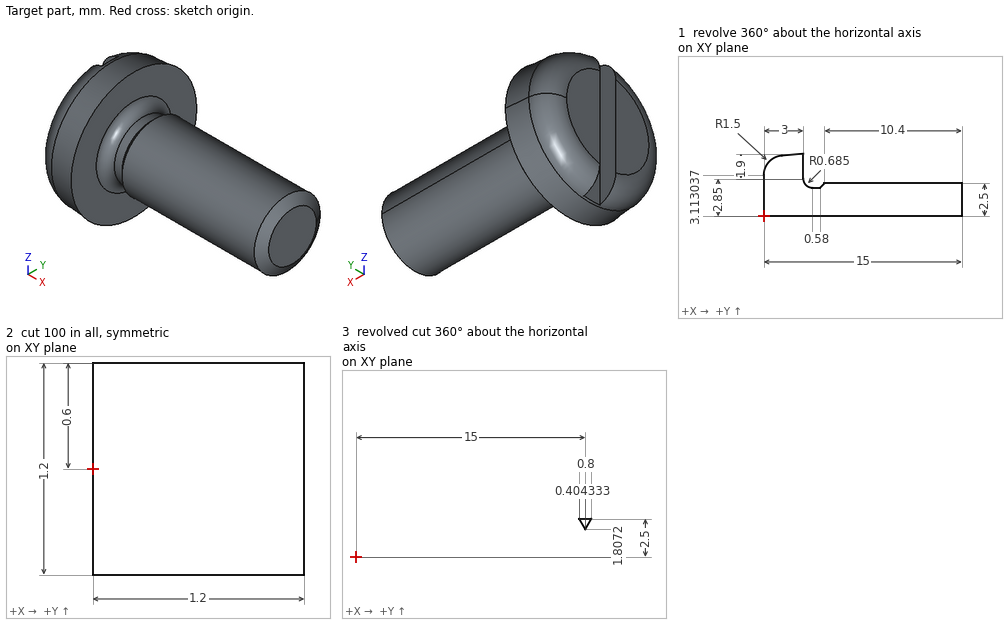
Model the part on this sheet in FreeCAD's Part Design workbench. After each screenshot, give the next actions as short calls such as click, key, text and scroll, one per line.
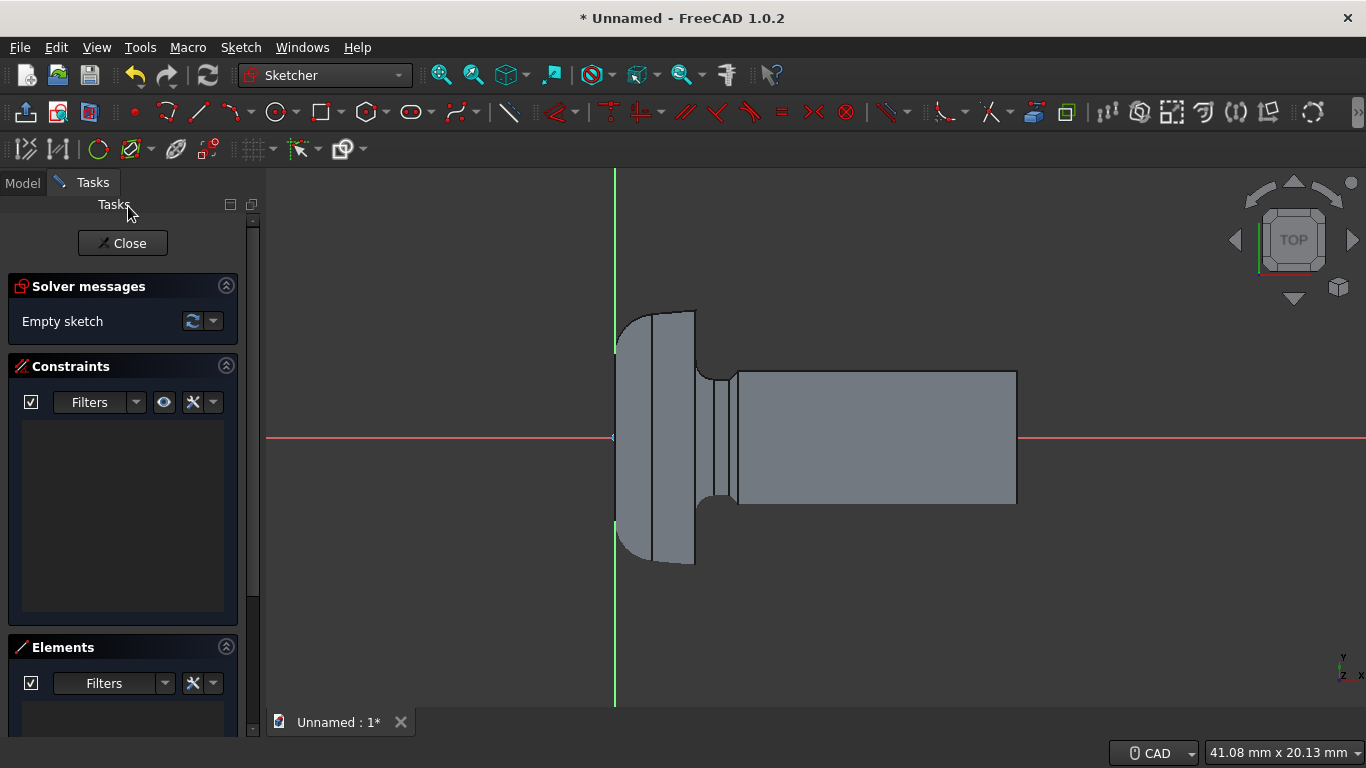
click(90, 112)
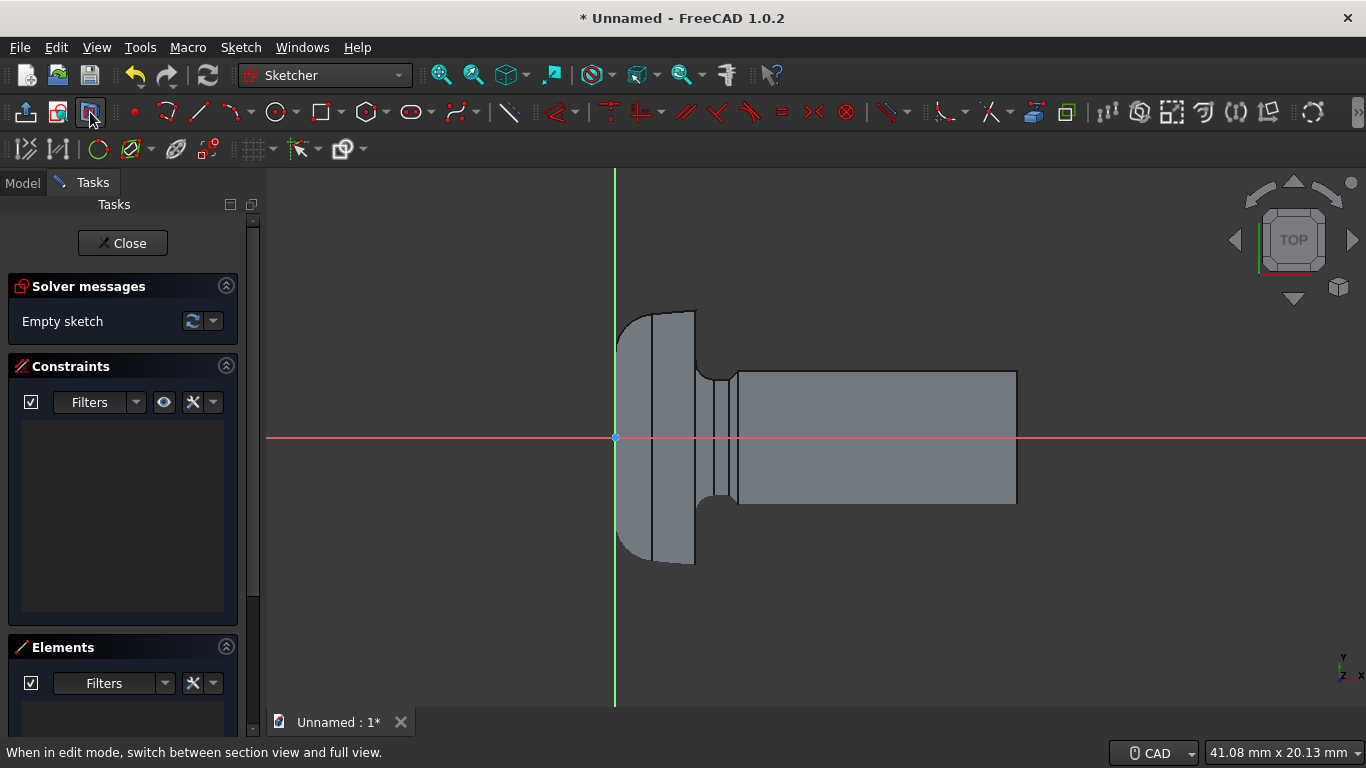
scroll(620, 438, up, 12)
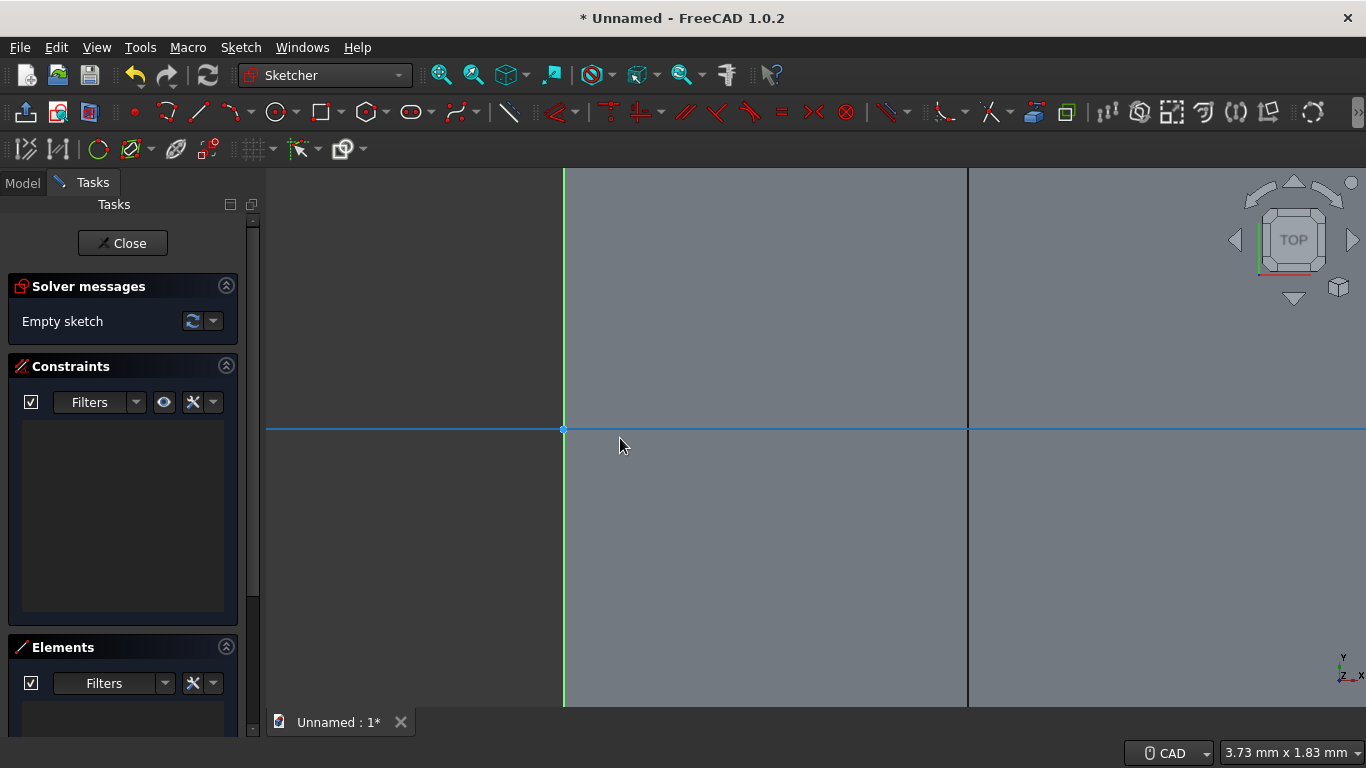
key(g)
key(r)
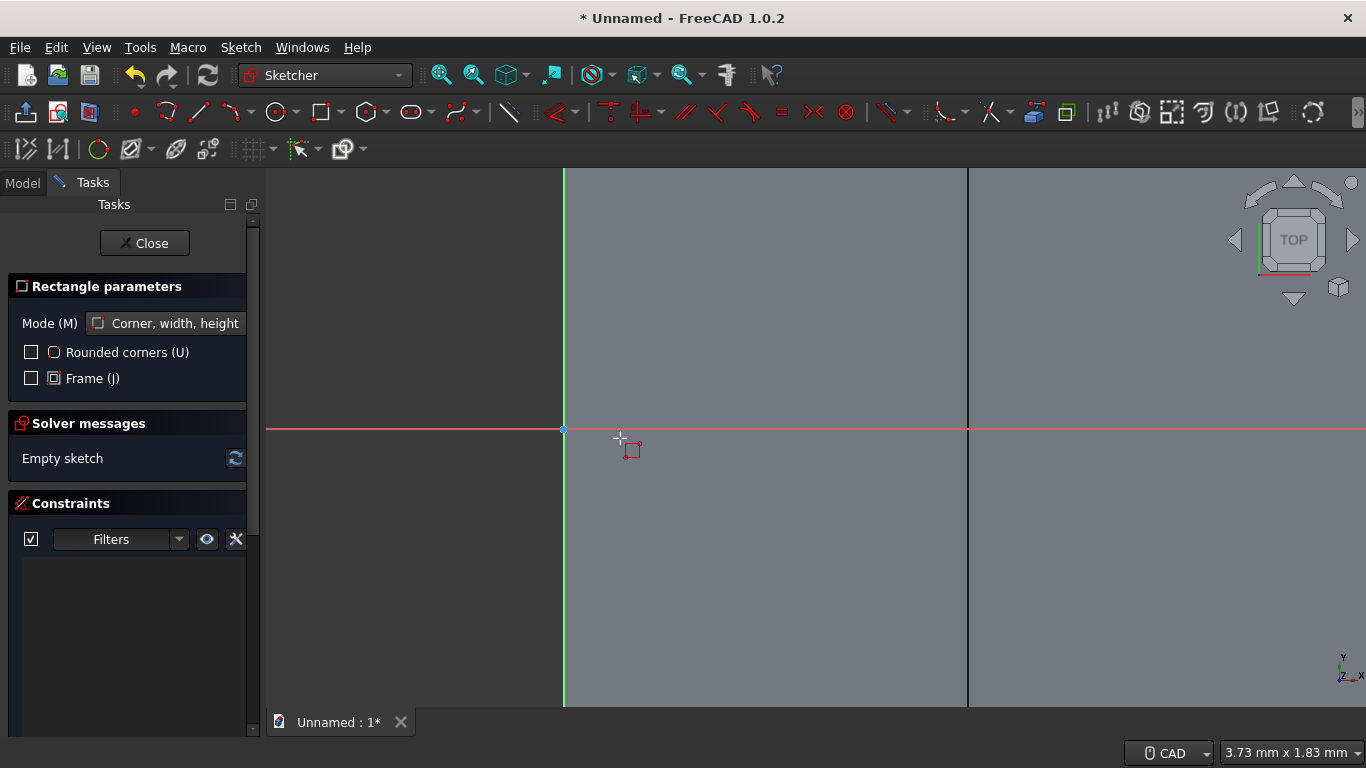
click(564, 252)
click(918, 606)
key(Escape)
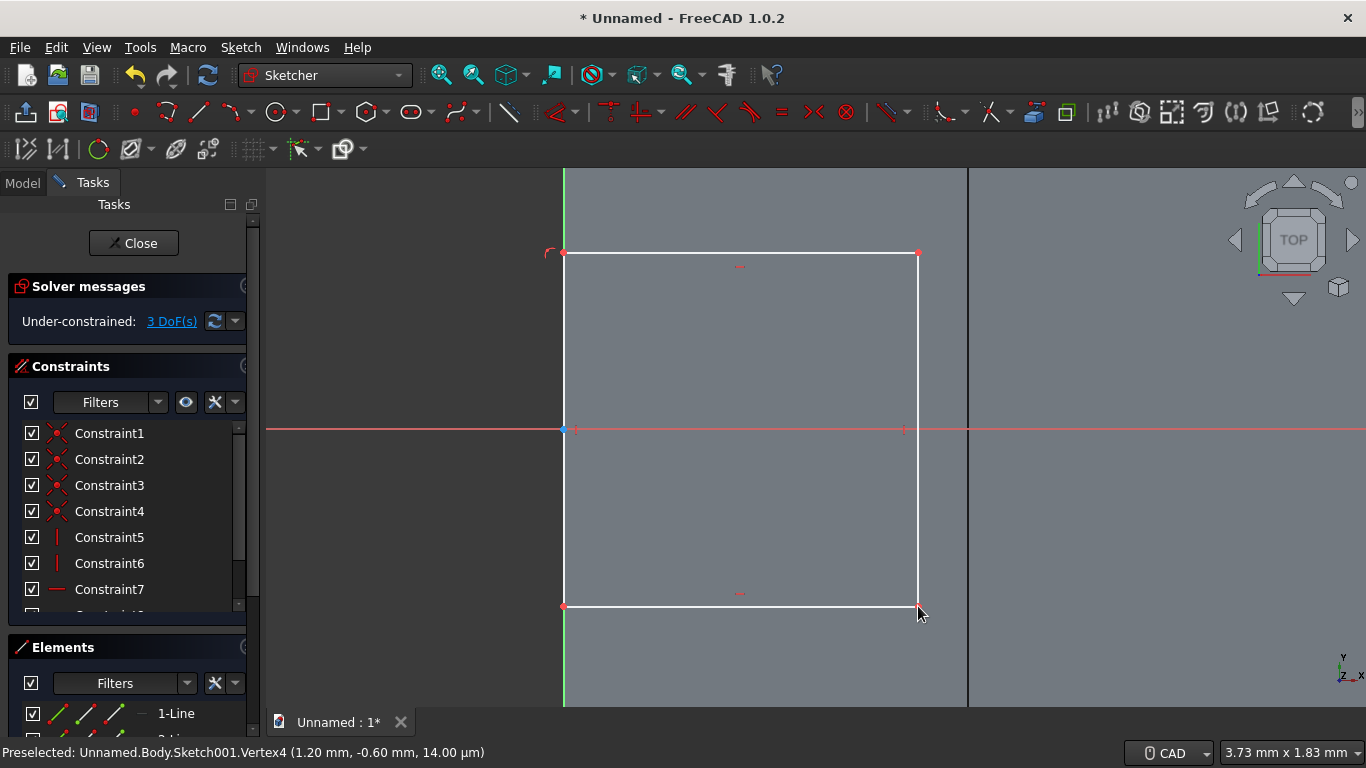
key(d)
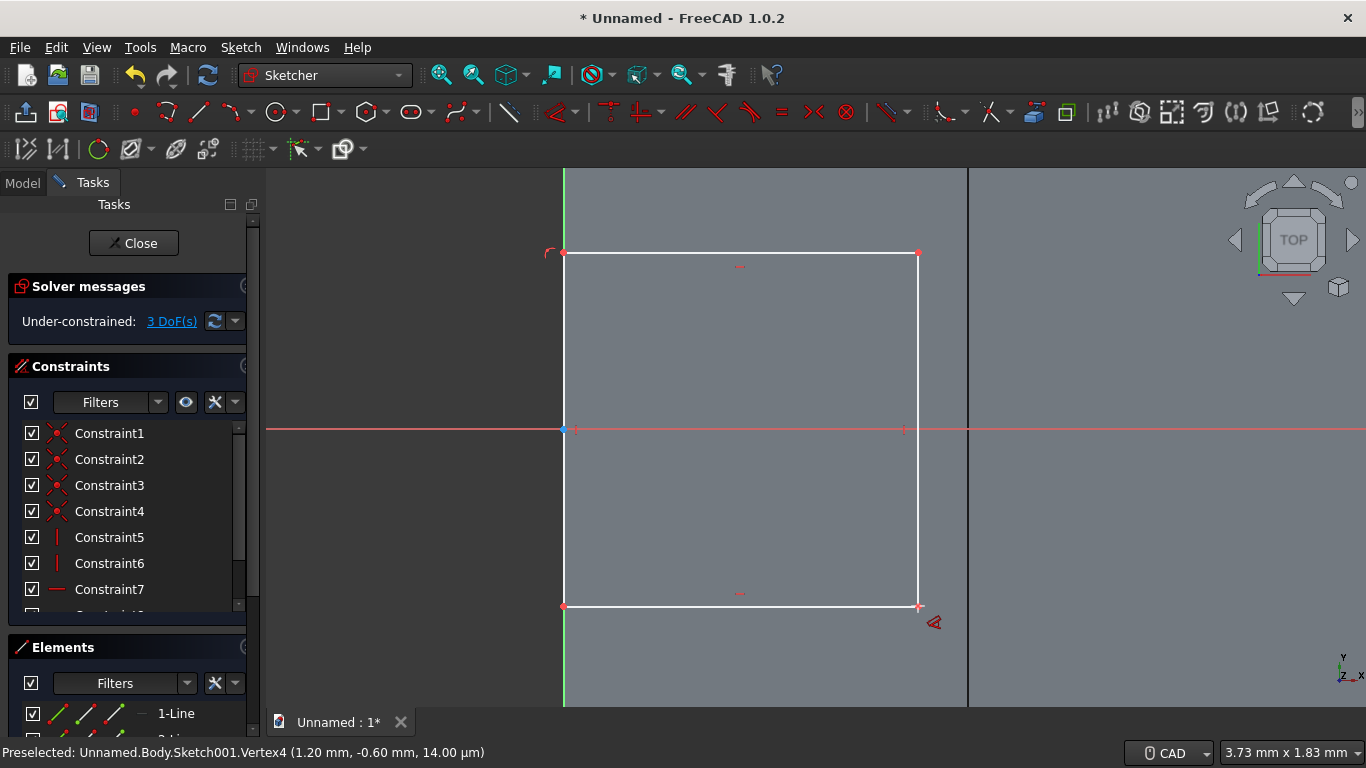
click(564, 359)
click(530, 349)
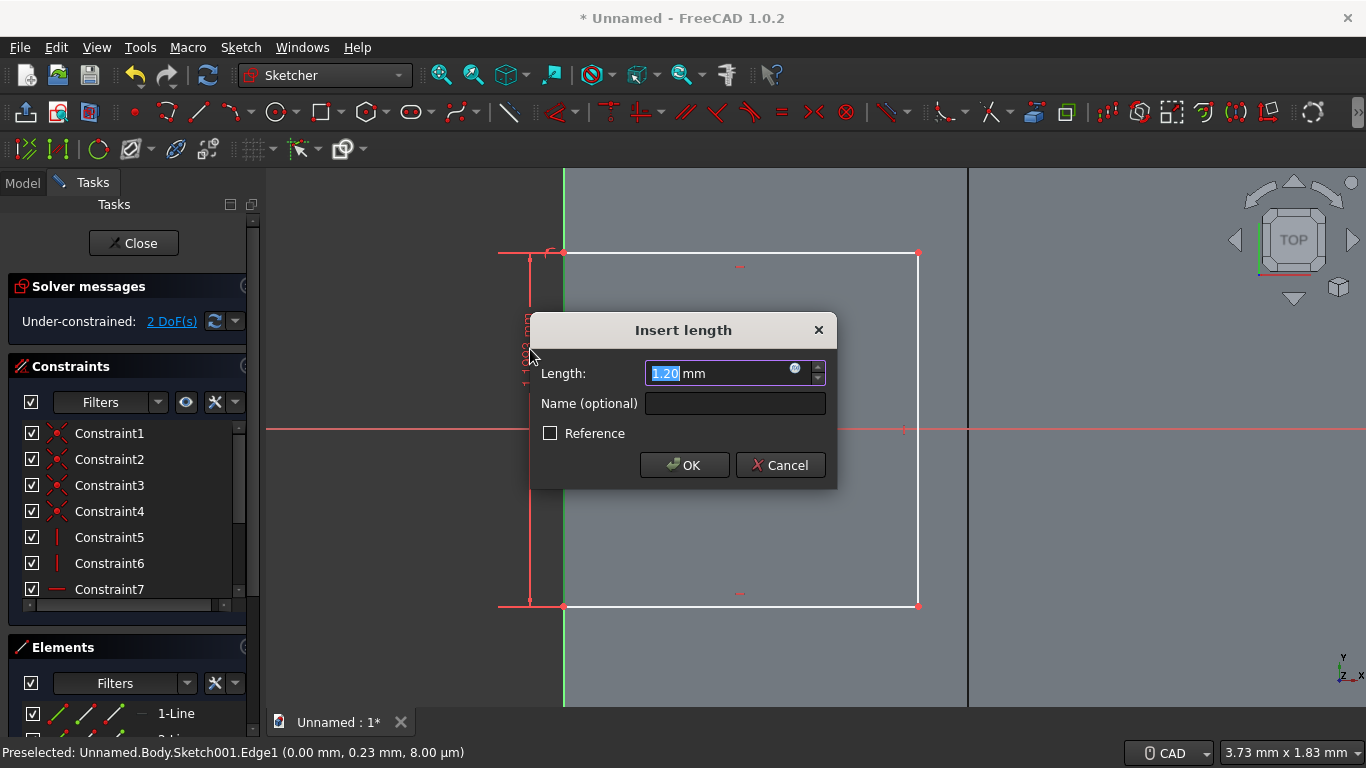
text(1.2)
key(Return)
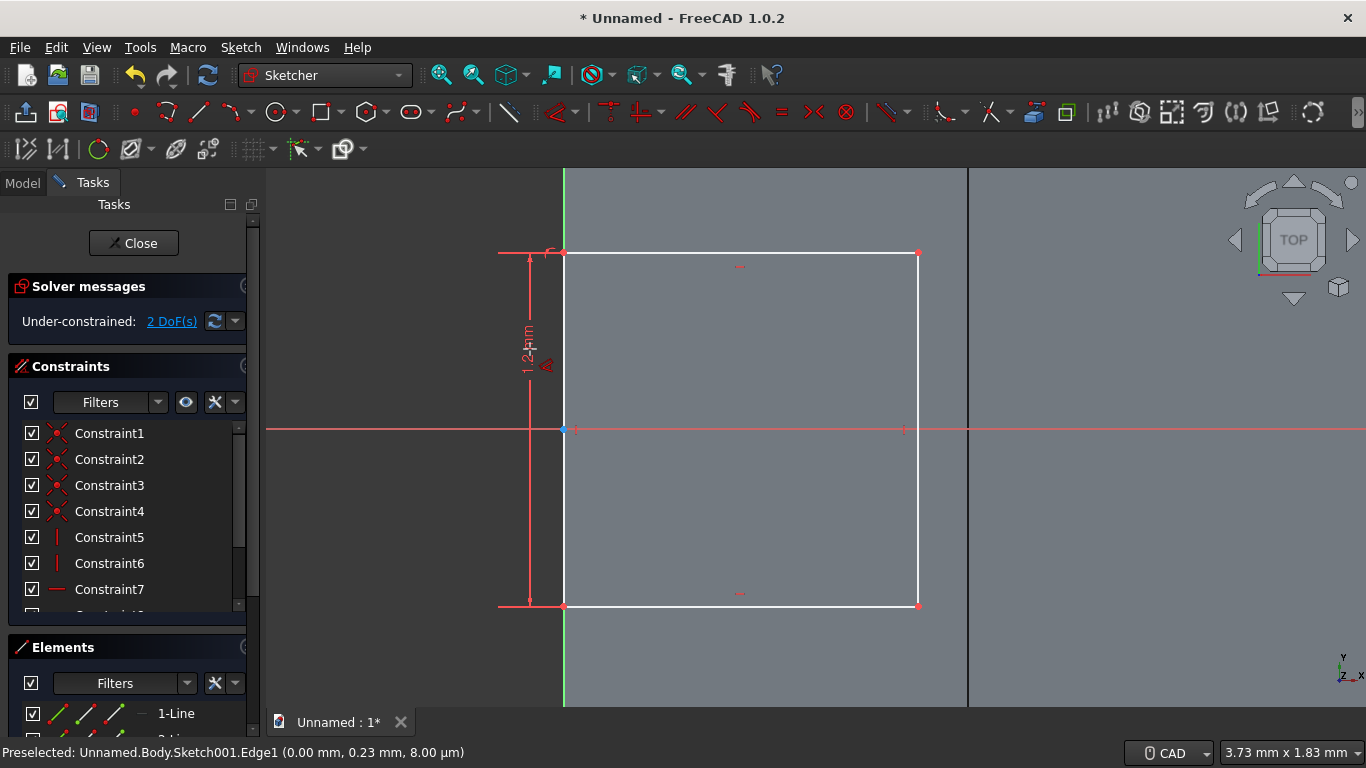
click(670, 607)
click(741, 641)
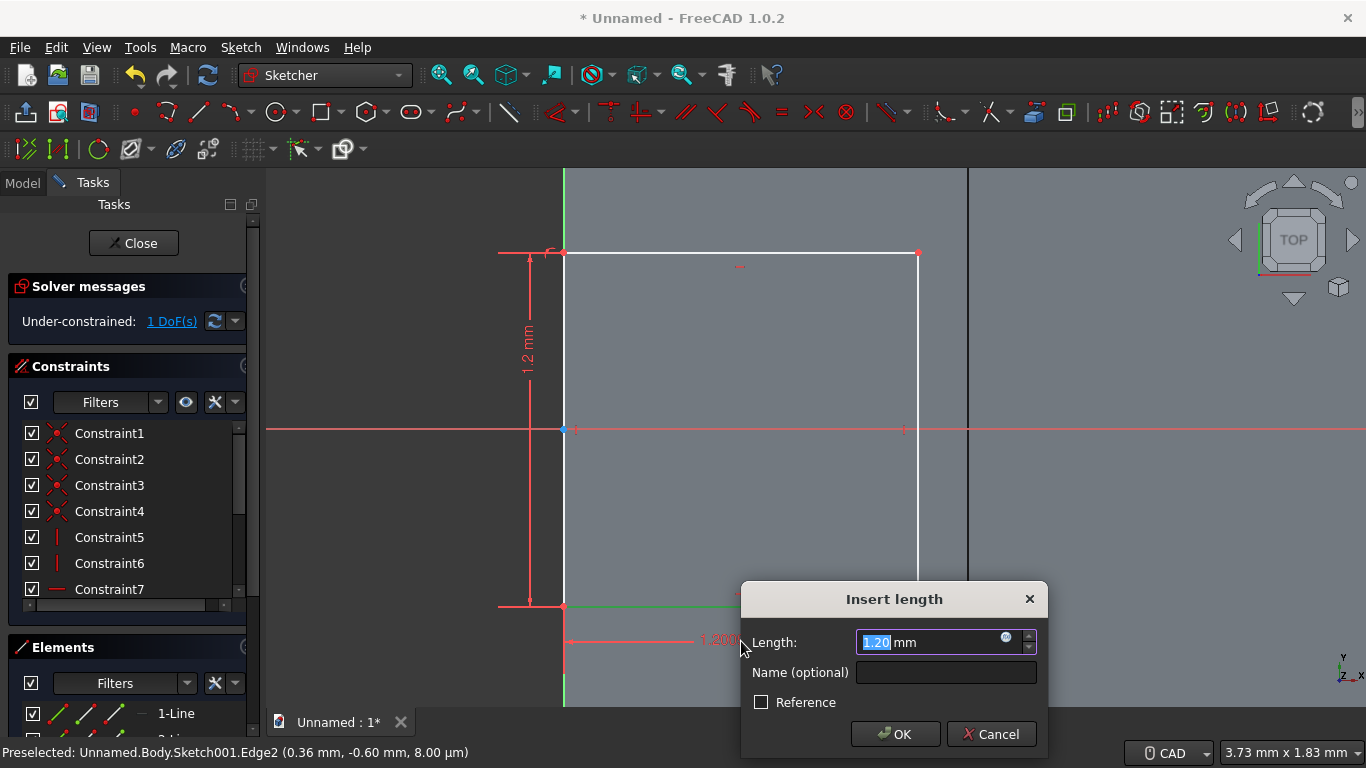
text(1.2)
key(Return)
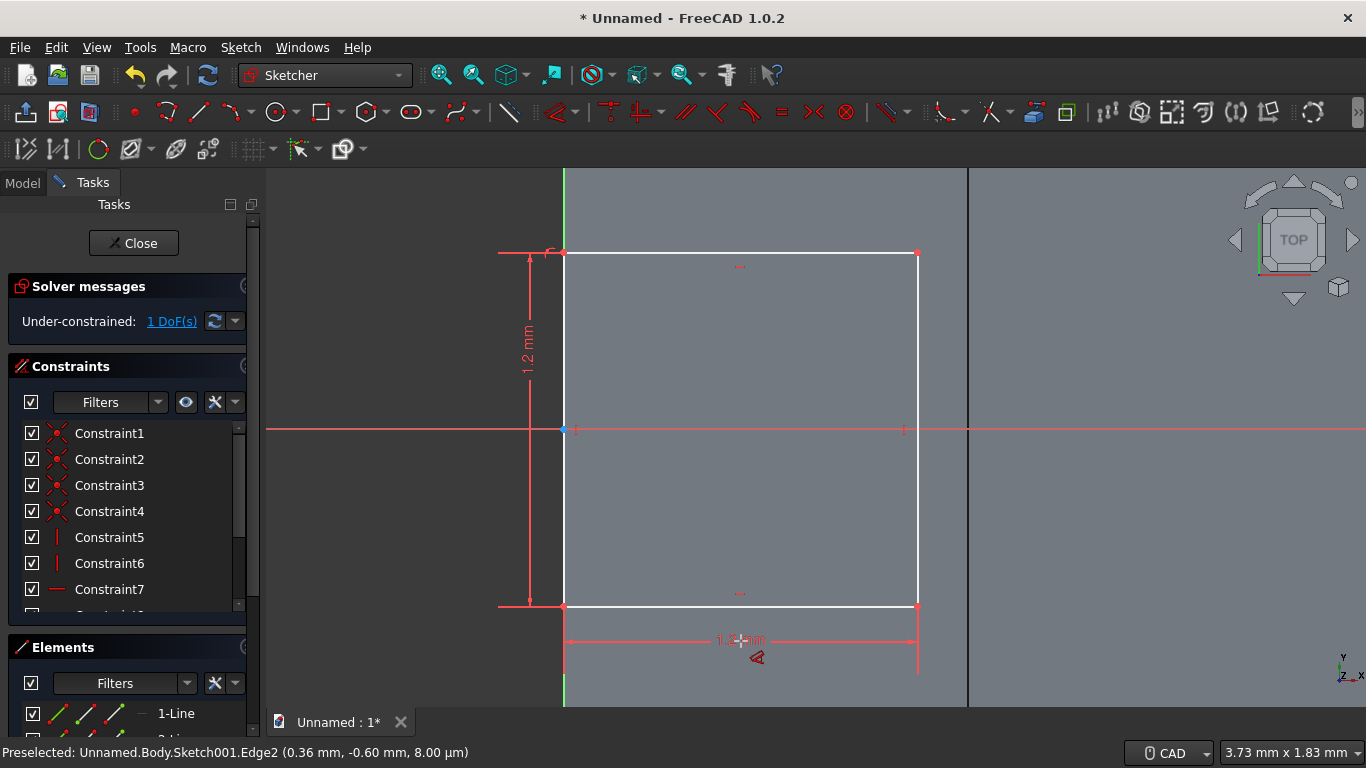
click(564, 253)
click(530, 300)